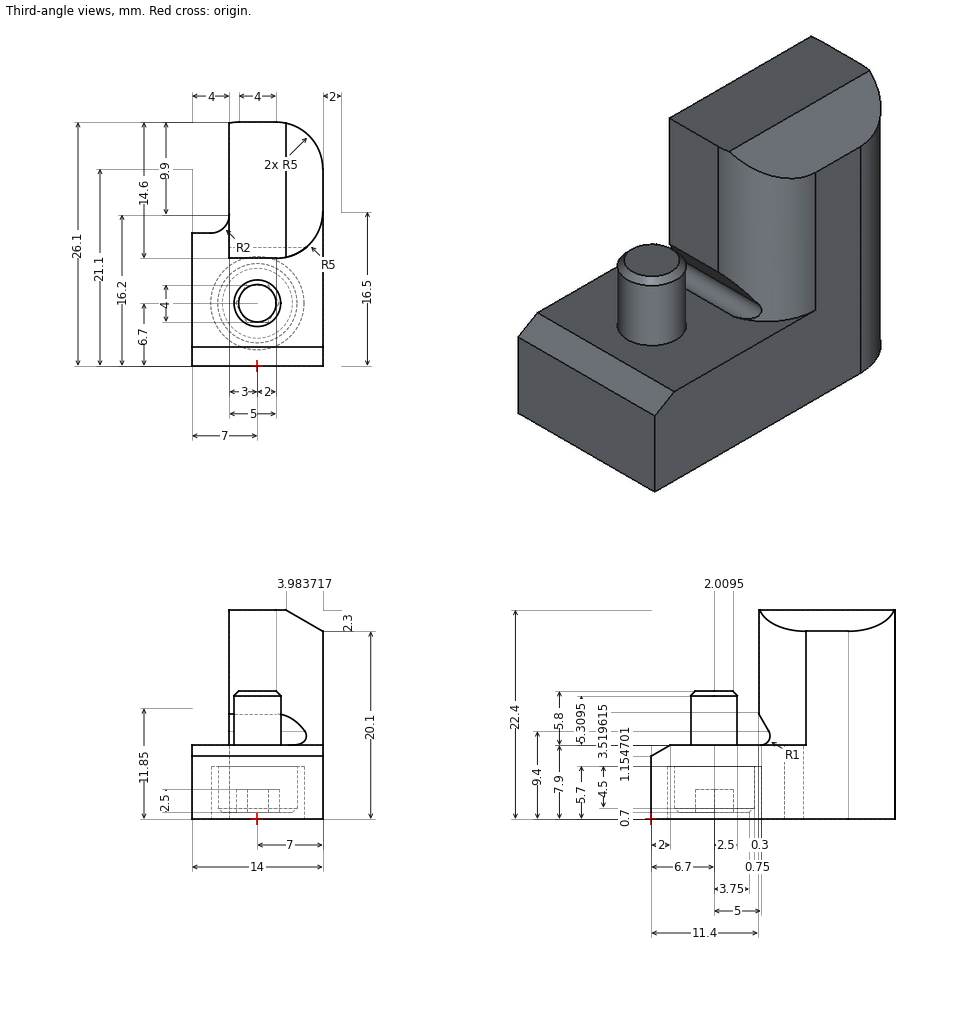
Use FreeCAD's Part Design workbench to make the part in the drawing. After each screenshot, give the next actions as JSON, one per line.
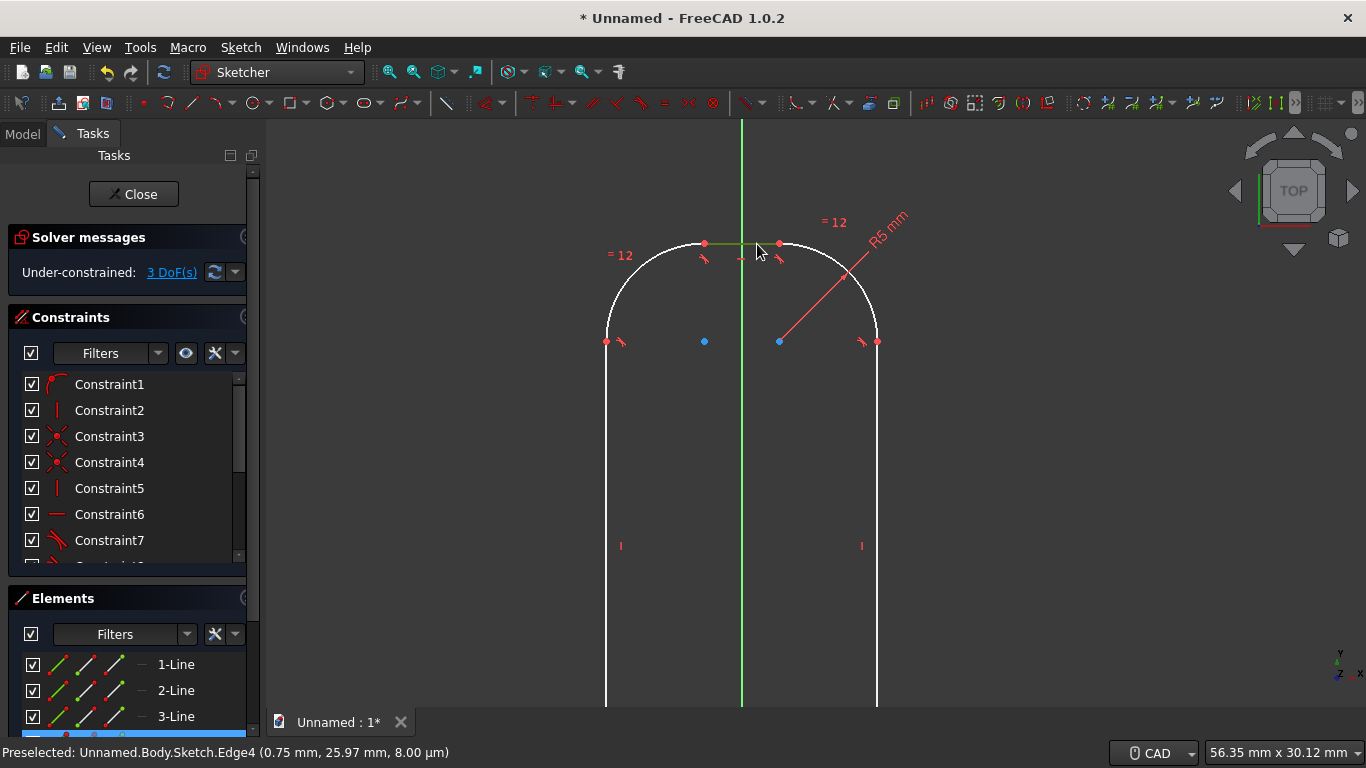
{"action": "left_click", "coordinate": [504, 104]}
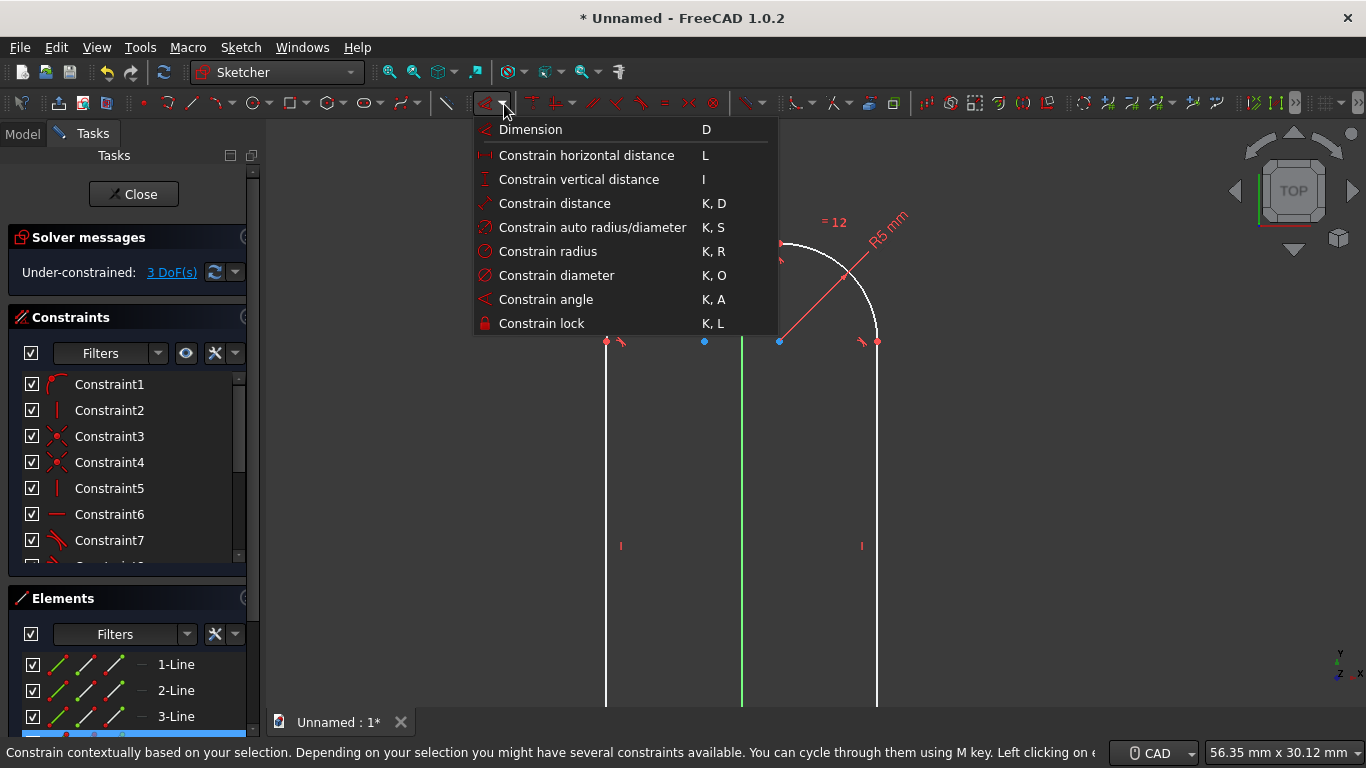
{"action": "left_click", "coordinate": [626, 155]}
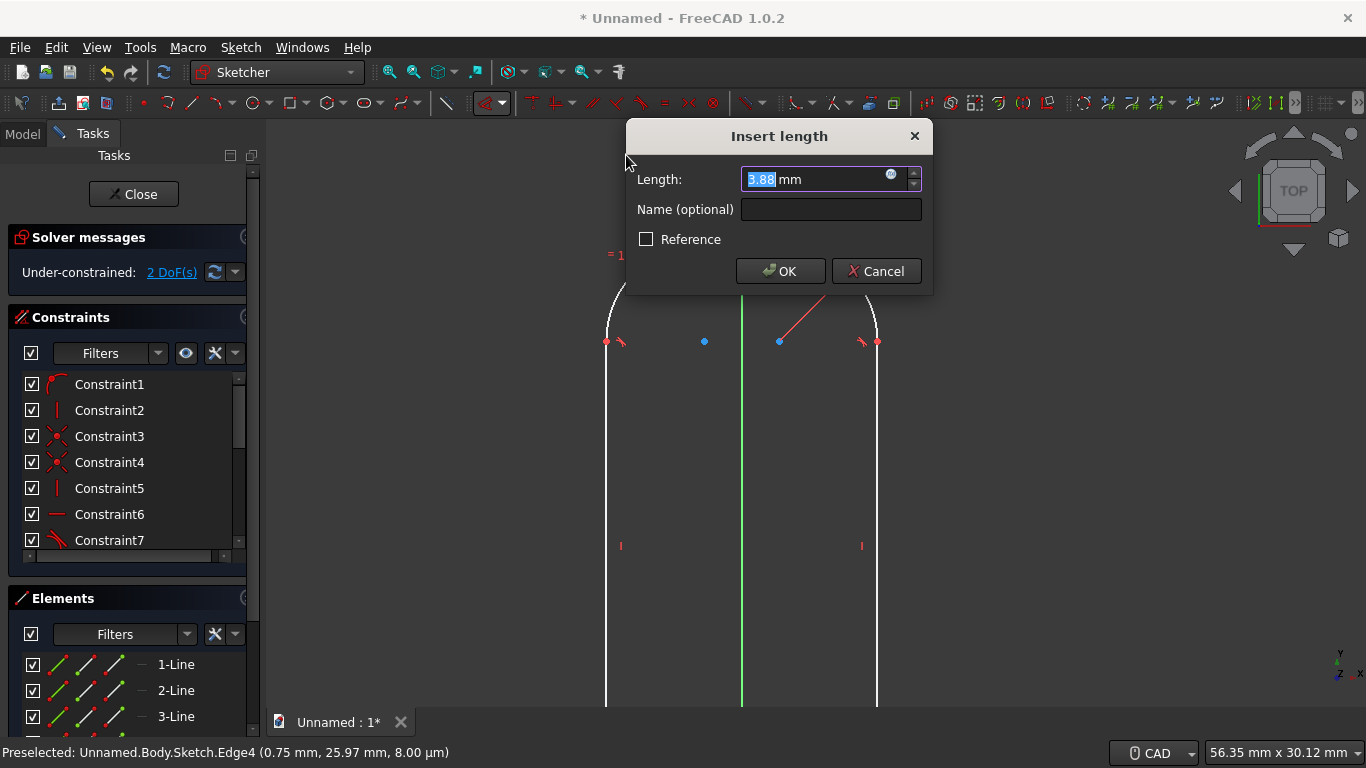
{"action": "type", "text": "4"}
{"action": "key", "text": "Return"}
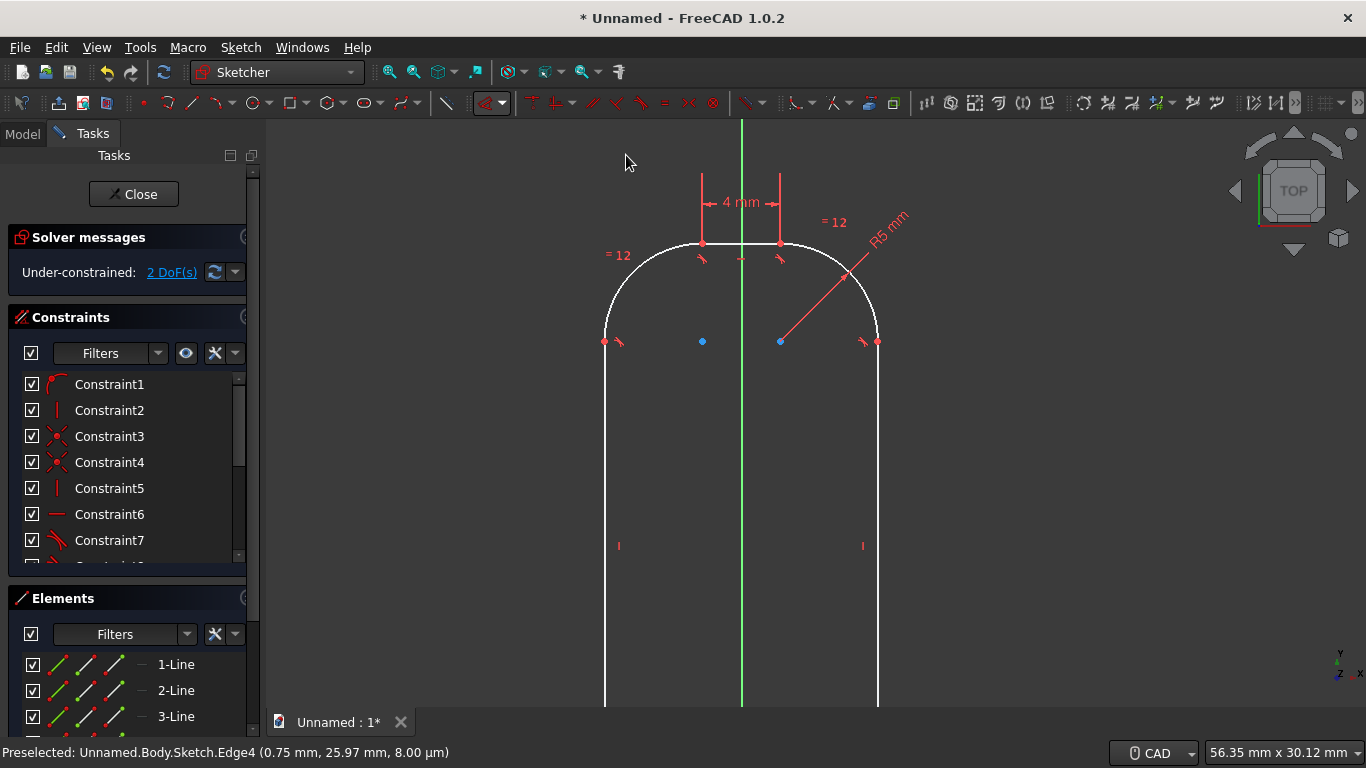
{"action": "left_click", "coordinate": [605, 341]}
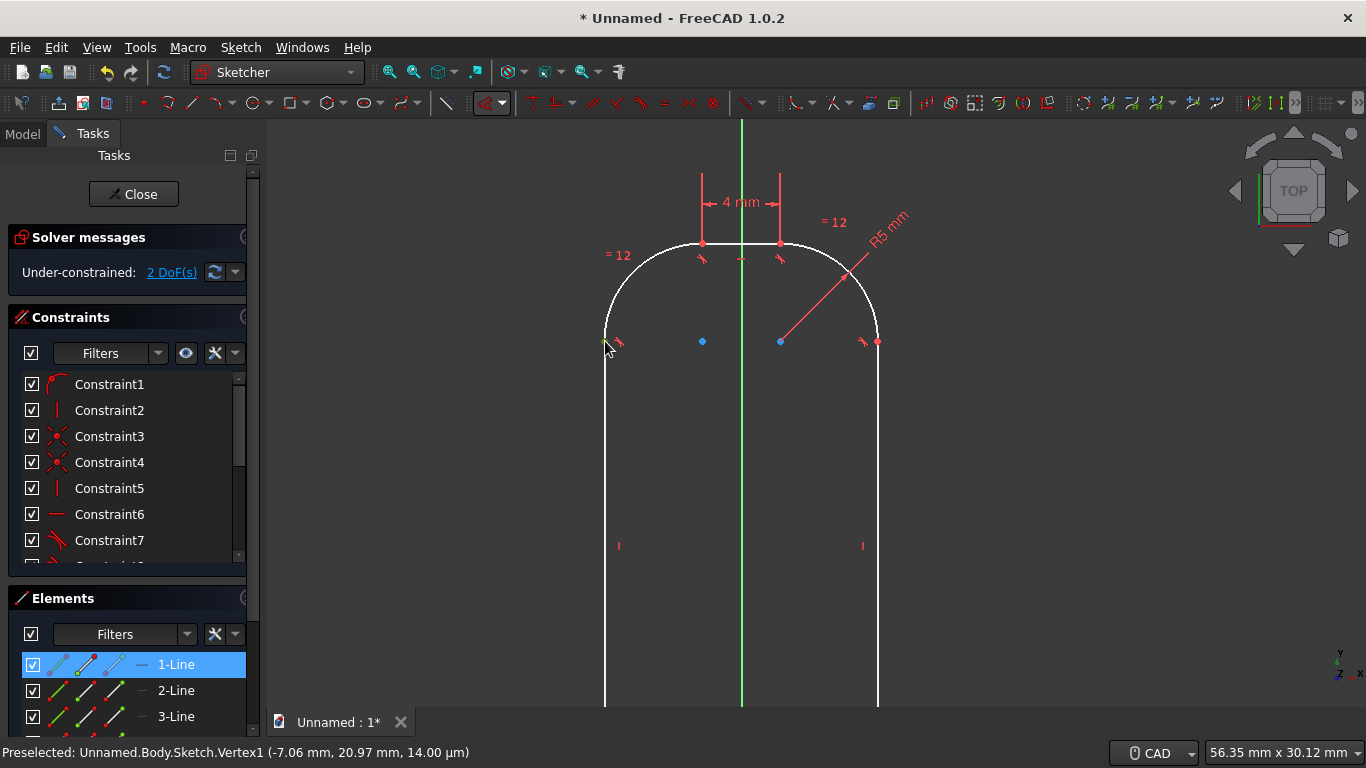
{"action": "key", "text": "l"}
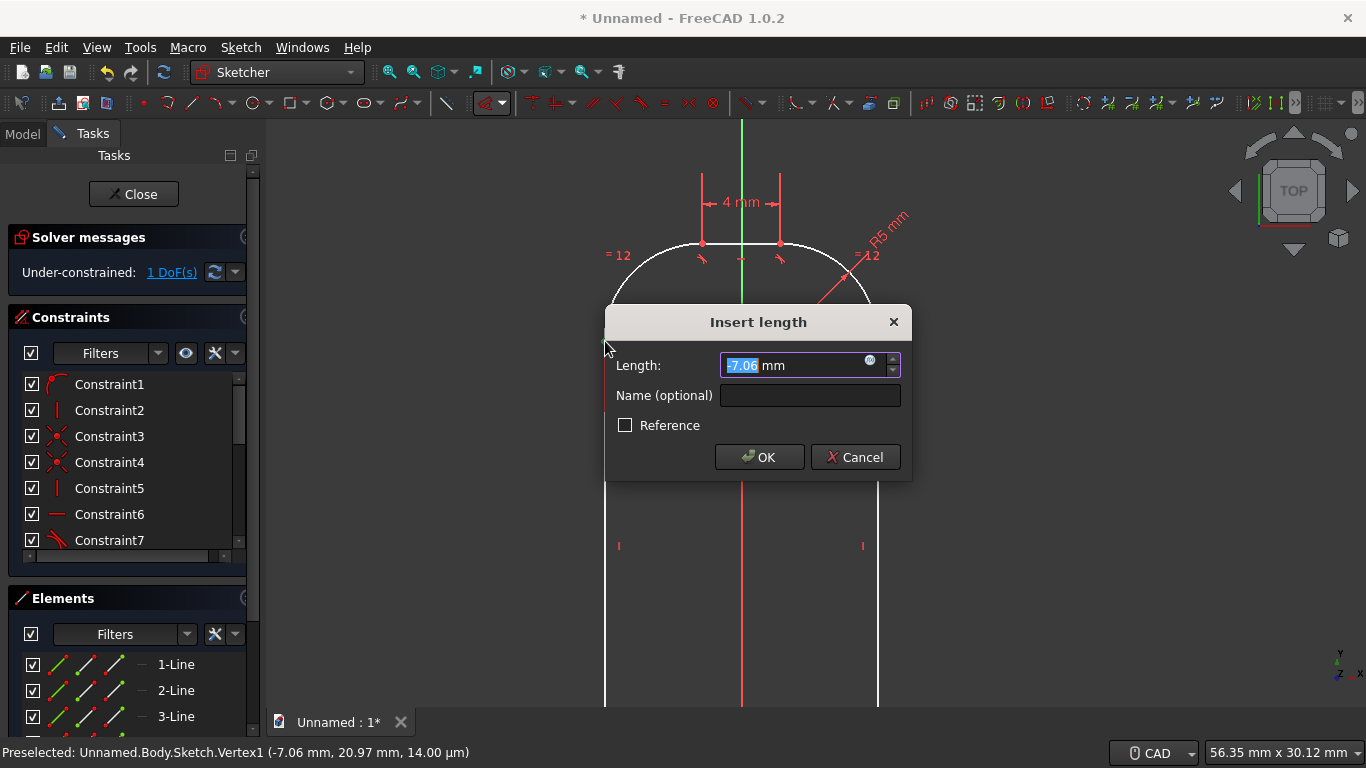
{"action": "type", "text": "-7"}
{"action": "key", "text": "Return"}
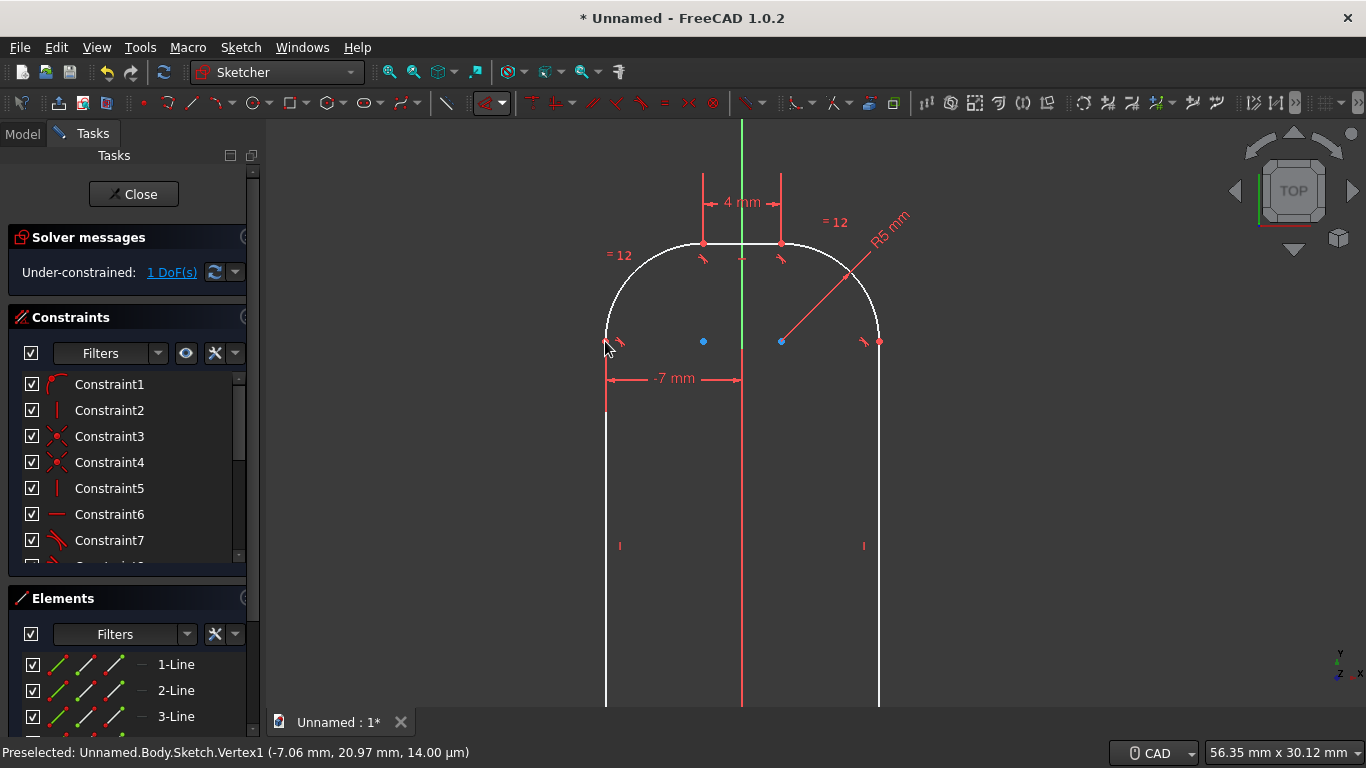
{"action": "left_click", "coordinate": [606, 464]}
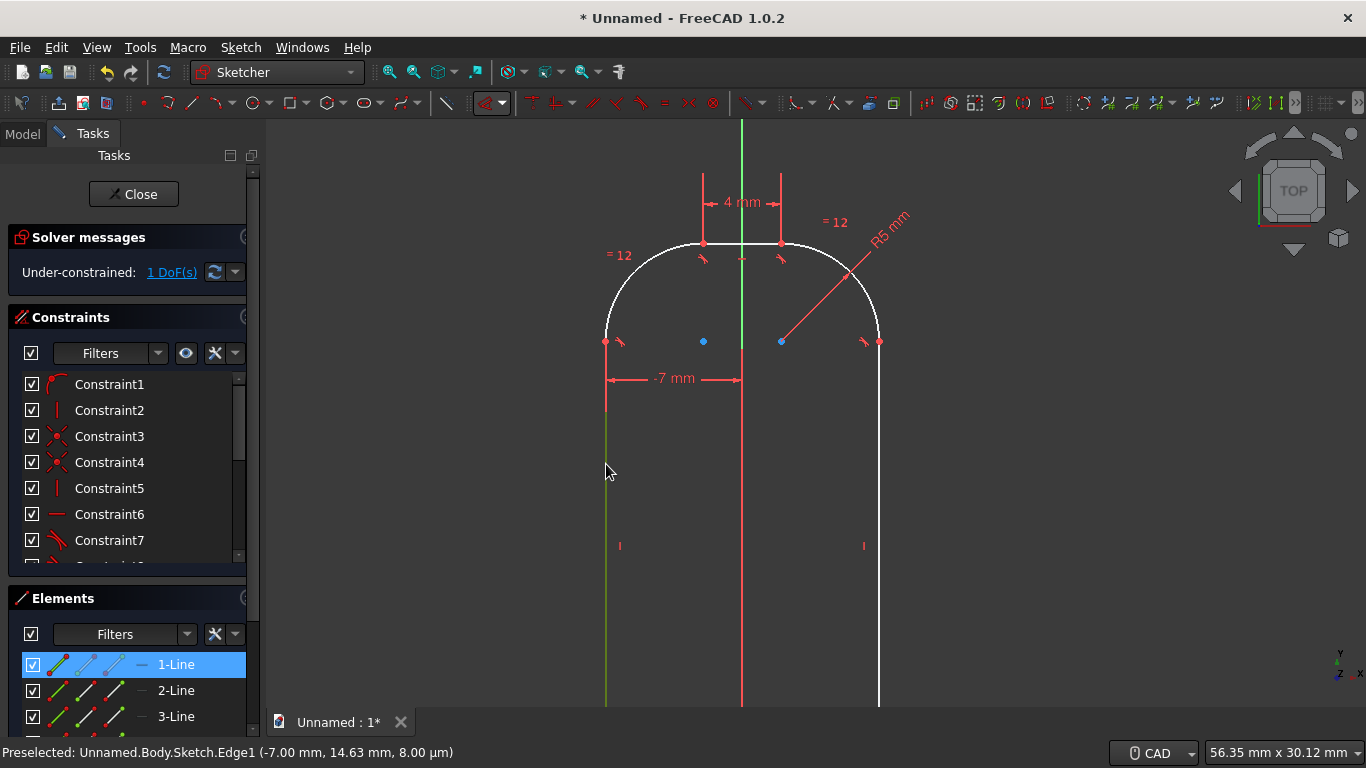
{"action": "left_click", "coordinate": [504, 104]}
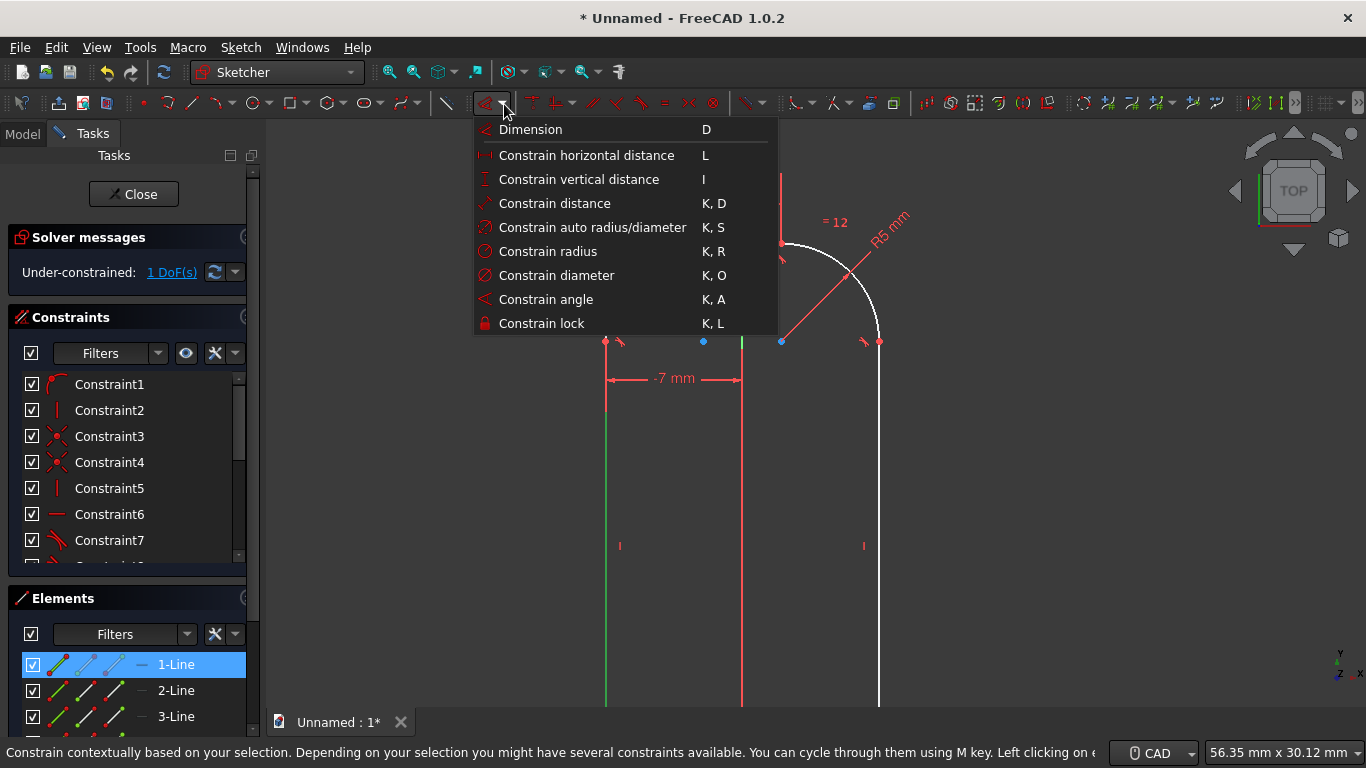
{"action": "left_click", "coordinate": [626, 179]}